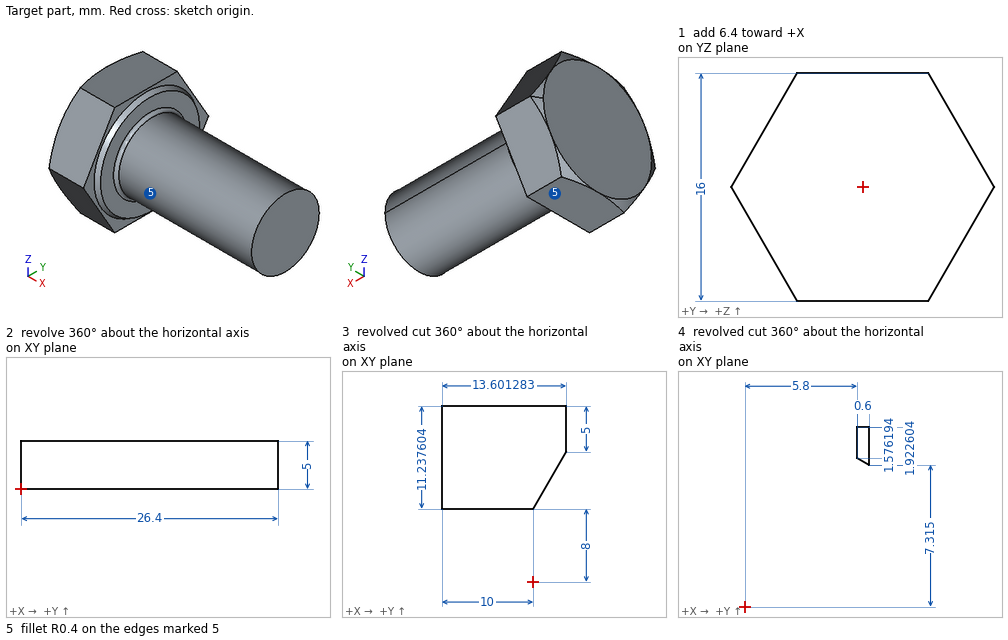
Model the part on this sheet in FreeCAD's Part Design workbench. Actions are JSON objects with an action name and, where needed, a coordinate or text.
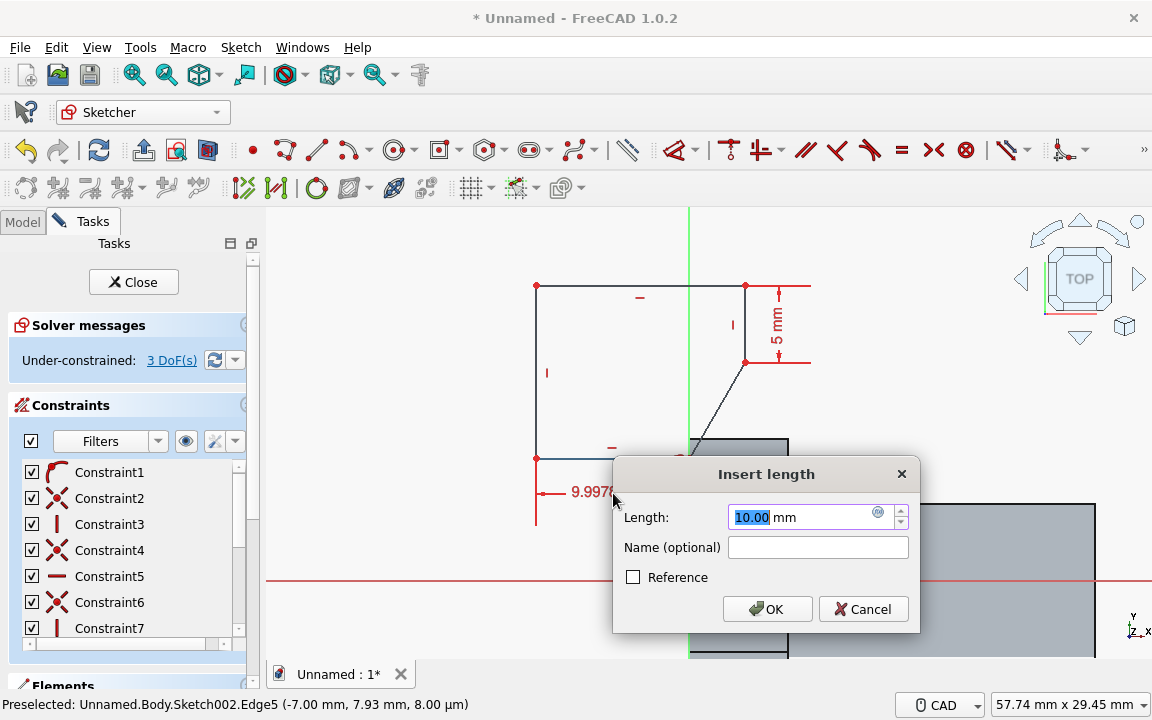
{"action": "type", "text": "10"}
{"action": "key", "text": "Return"}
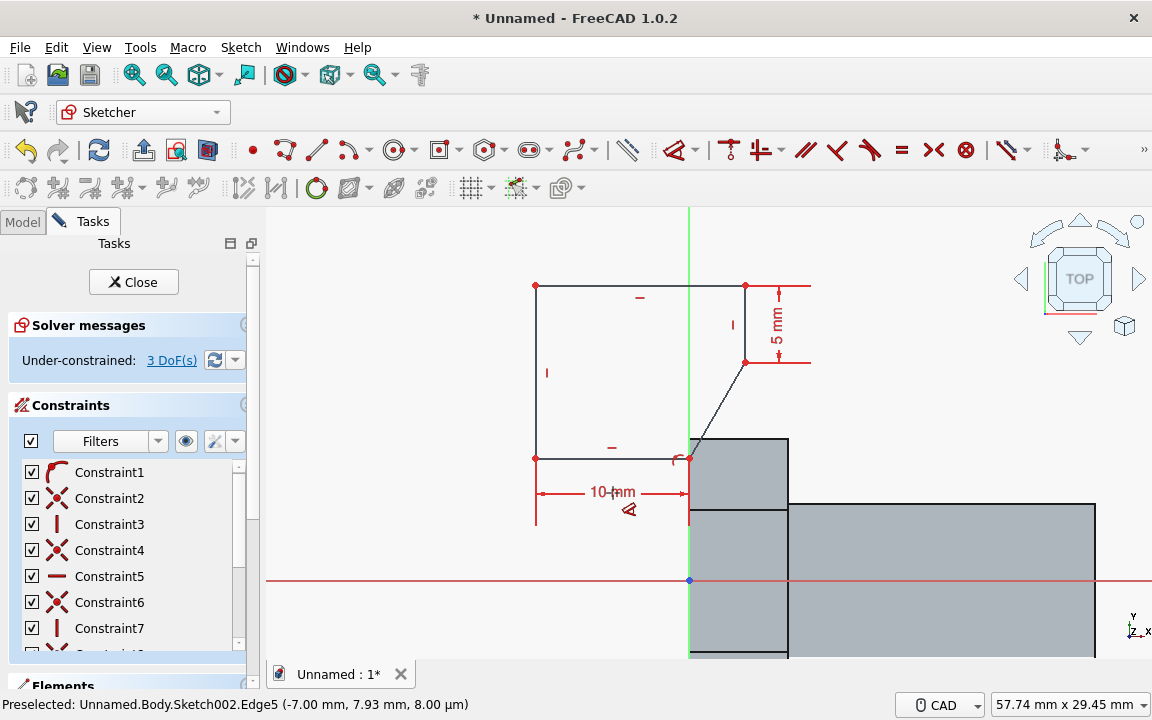
{"action": "left_click", "coordinate": [689, 459]}
{"action": "left_click", "coordinate": [723, 520]}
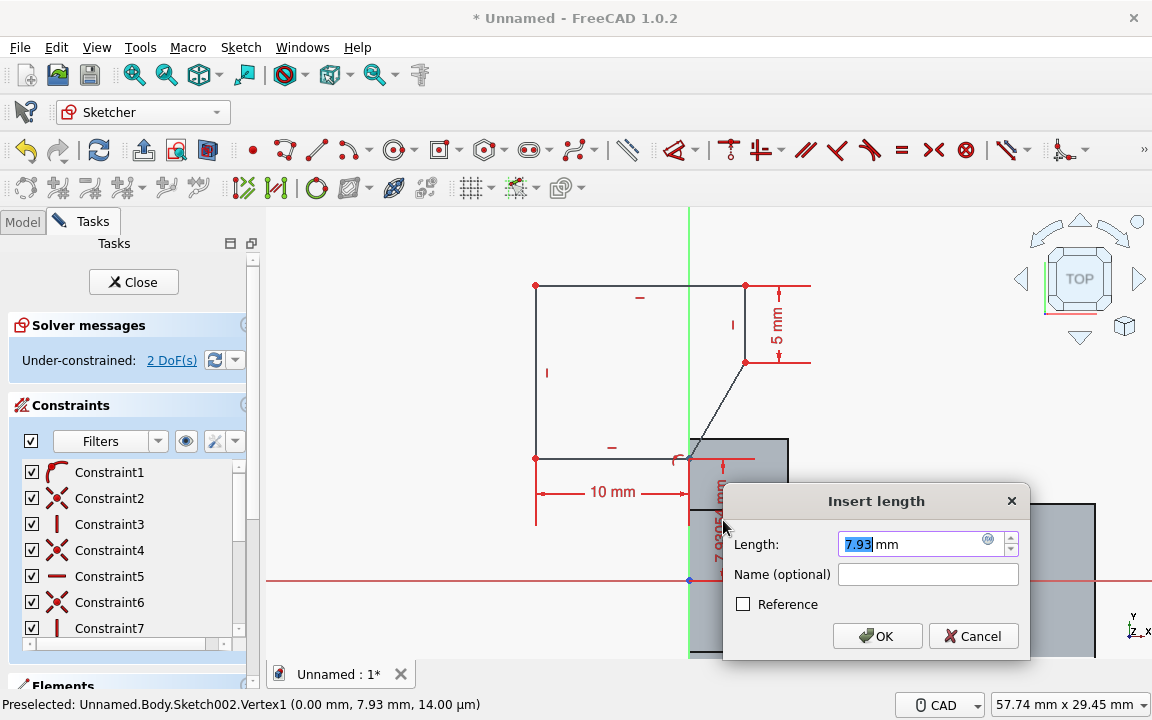
{"action": "type", "text": "8"}
{"action": "key", "text": "Return"}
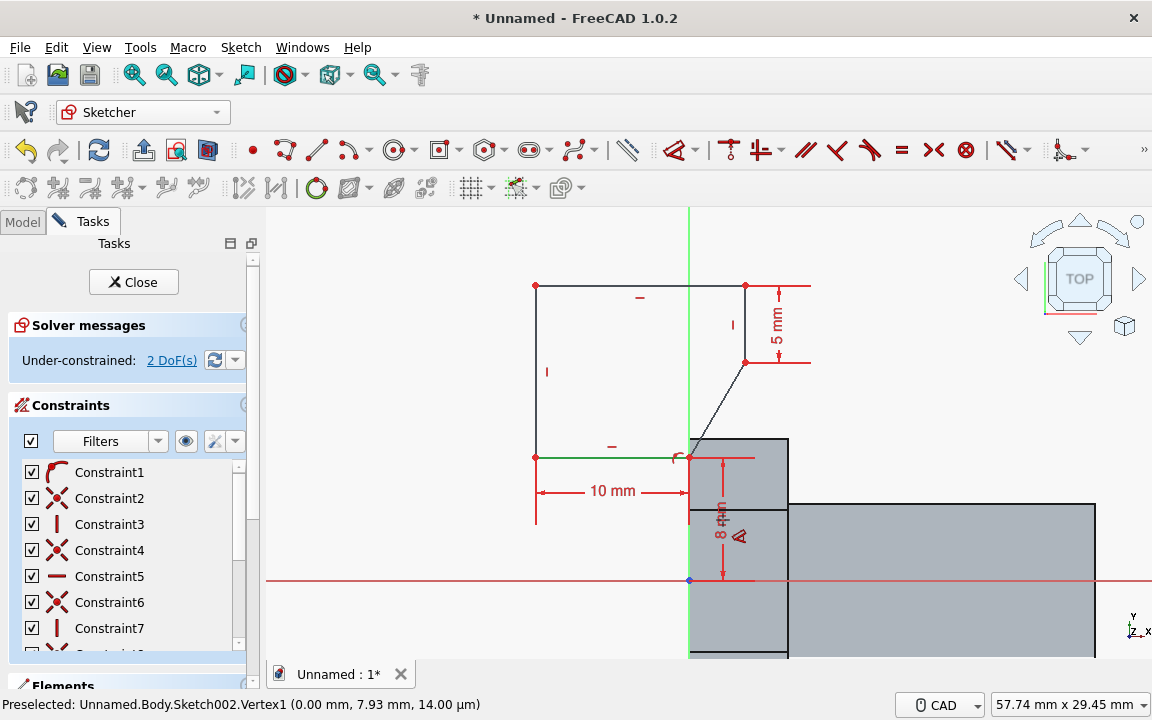
{"action": "left_click", "coordinate": [599, 286]}
{"action": "left_click", "coordinate": [640, 252]}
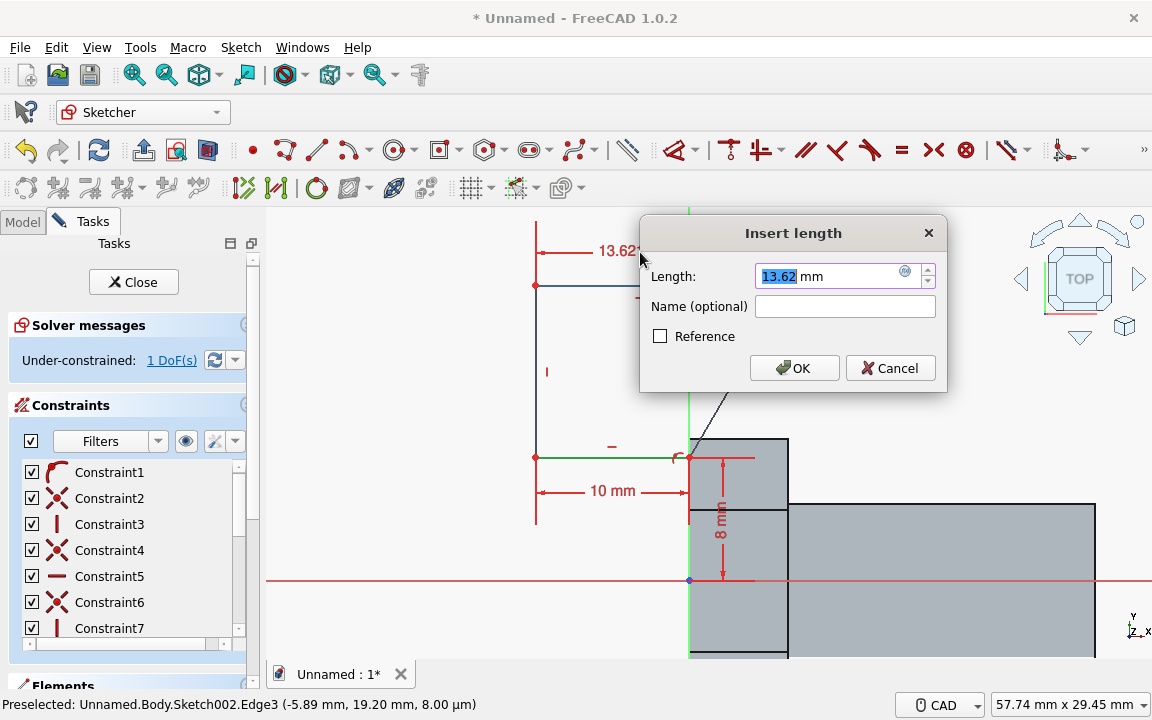
{"action": "type", "text": "13.601283"}
{"action": "key", "text": "Return"}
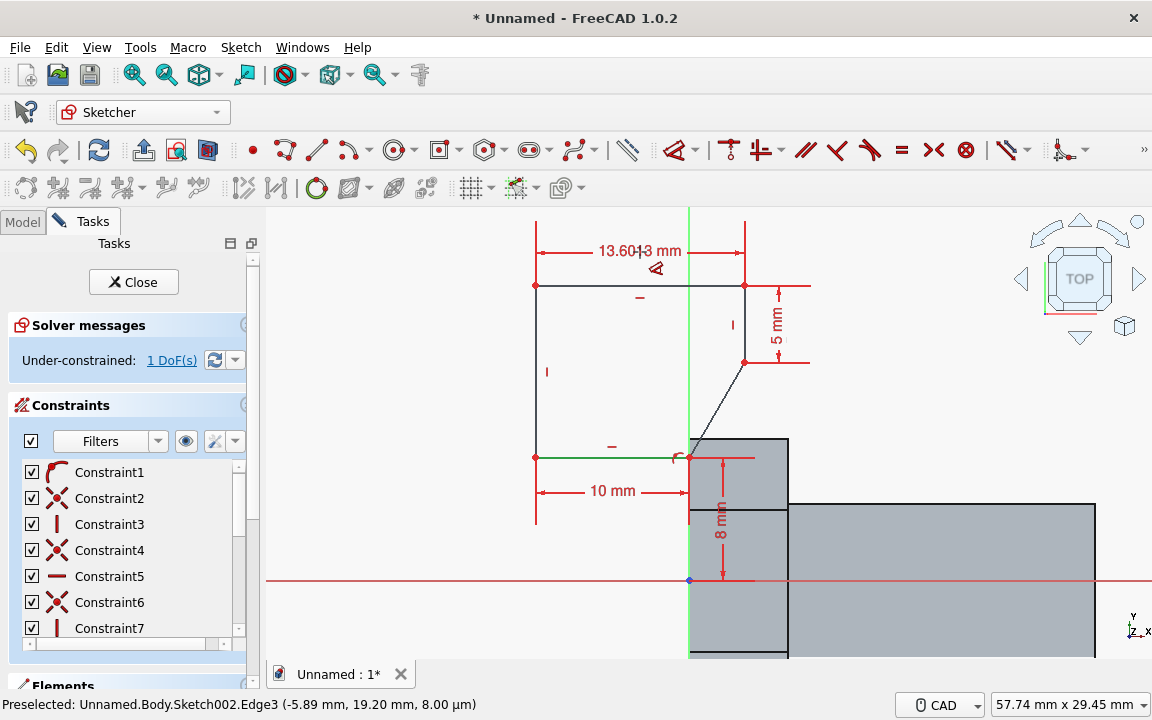
{"action": "left_click", "coordinate": [536, 338]}
{"action": "left_click", "coordinate": [502, 372]}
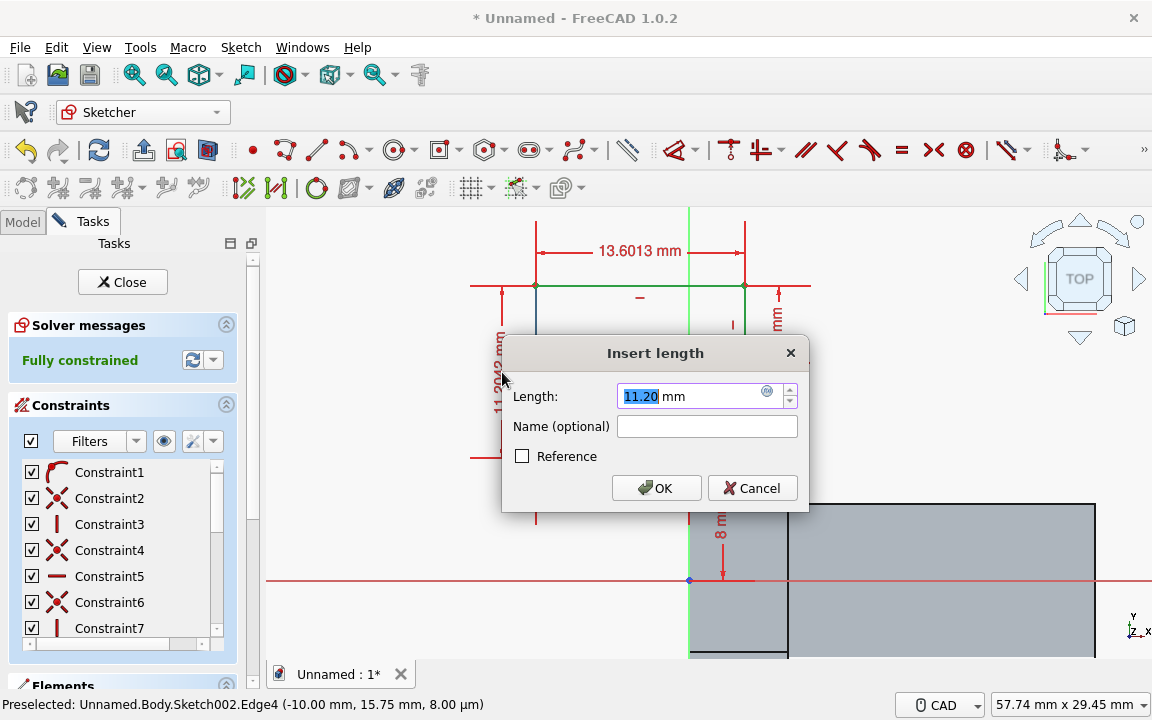
{"action": "type", "text": "11.237604"}
{"action": "key", "text": "Return"}
{"action": "key", "text": "Escape"}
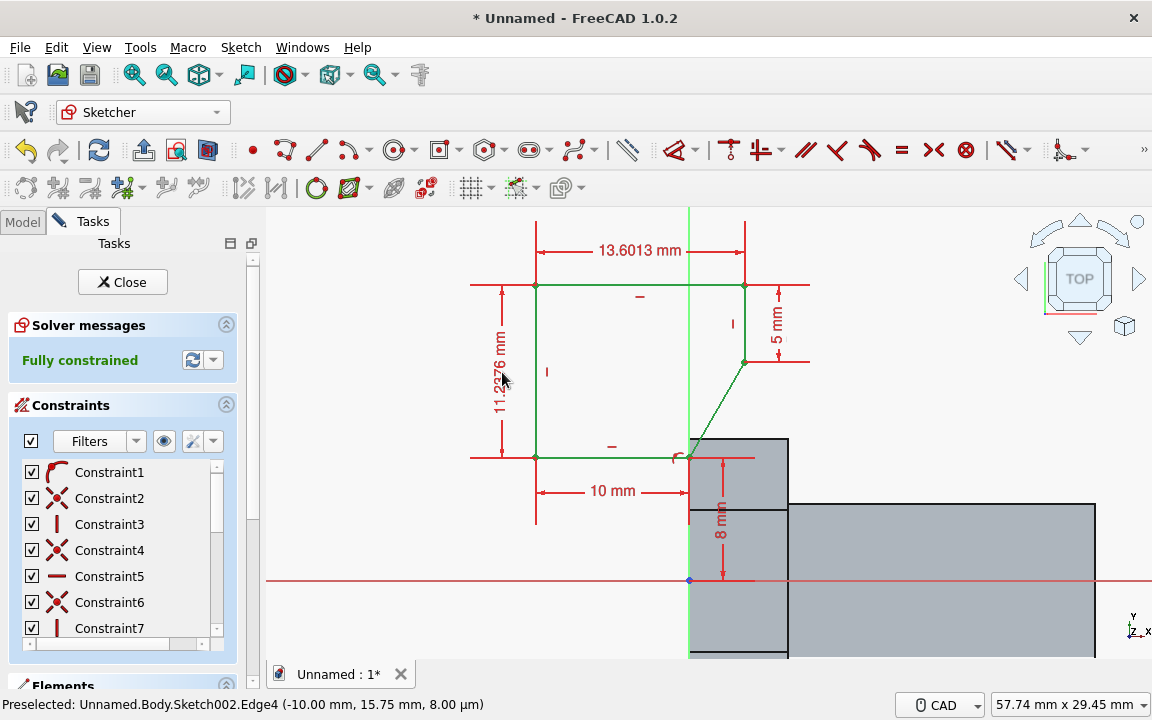
{"action": "left_click", "coordinate": [123, 282]}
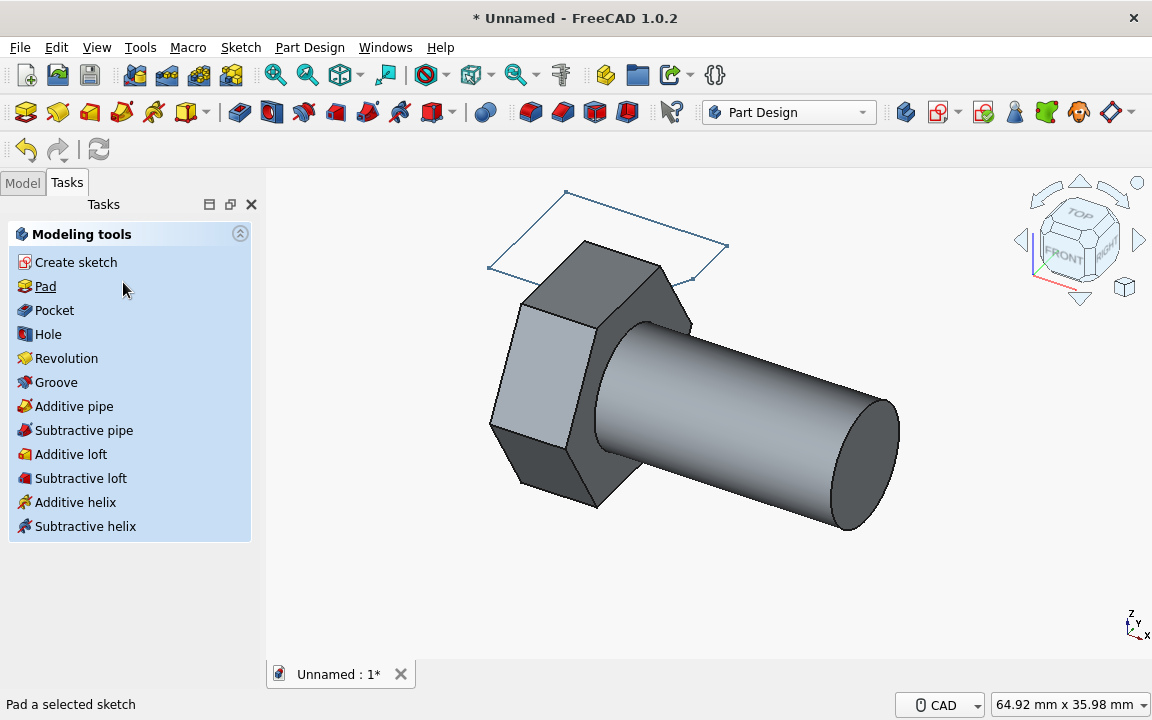
{"action": "left_click", "coordinate": [304, 112]}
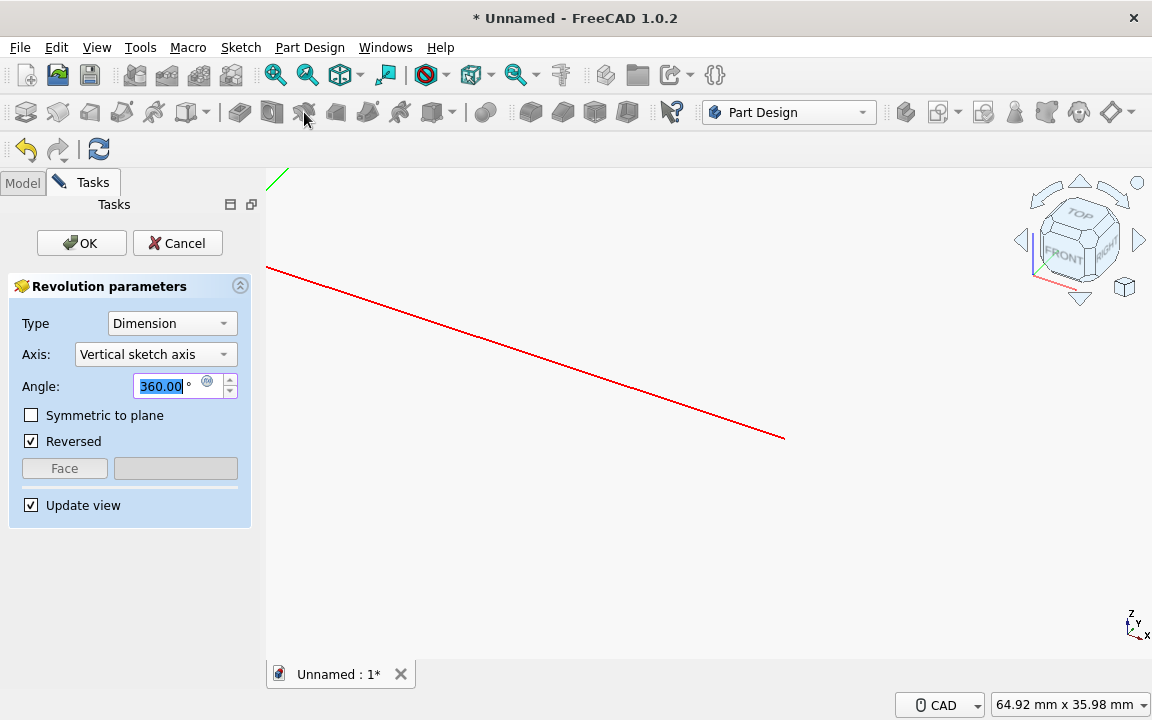
{"action": "left_click", "coordinate": [156, 354]}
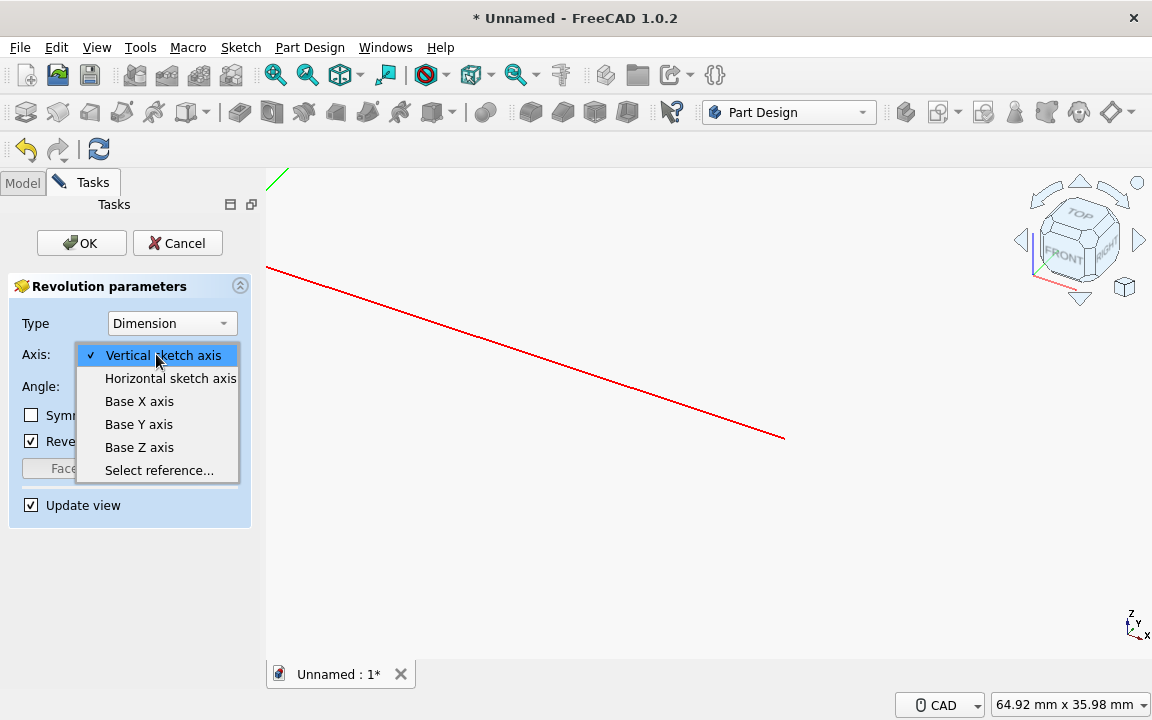
{"action": "left_click", "coordinate": [156, 378]}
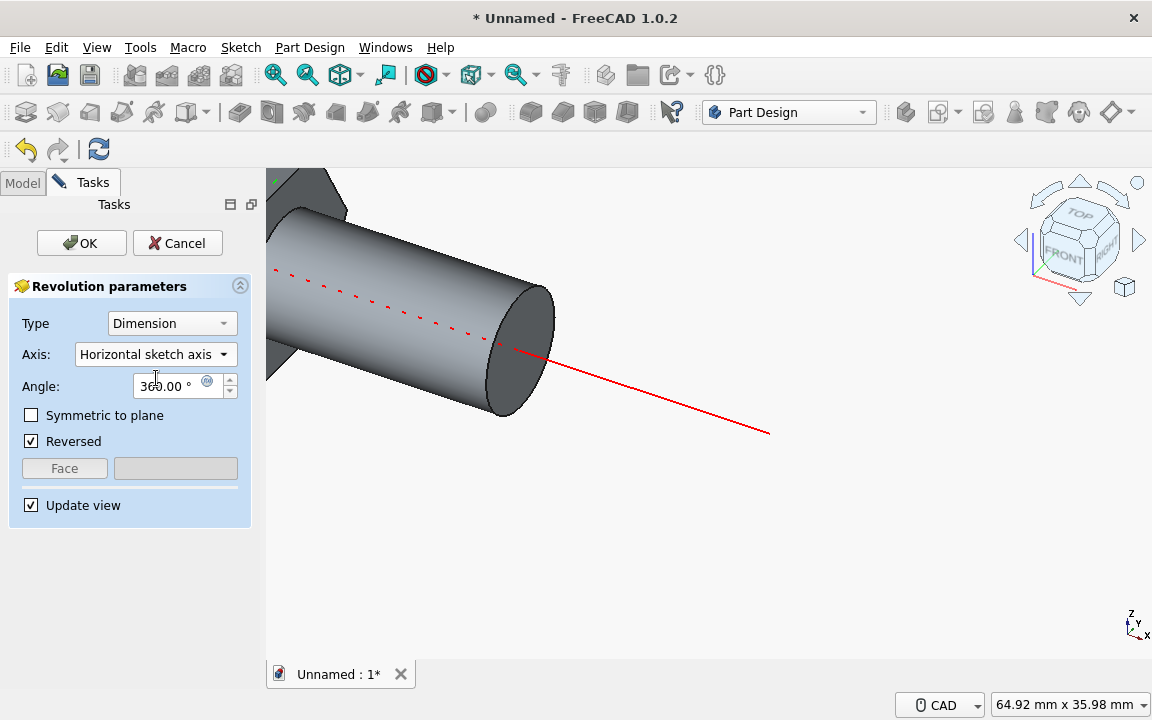
{"action": "left_click", "coordinate": [82, 243]}